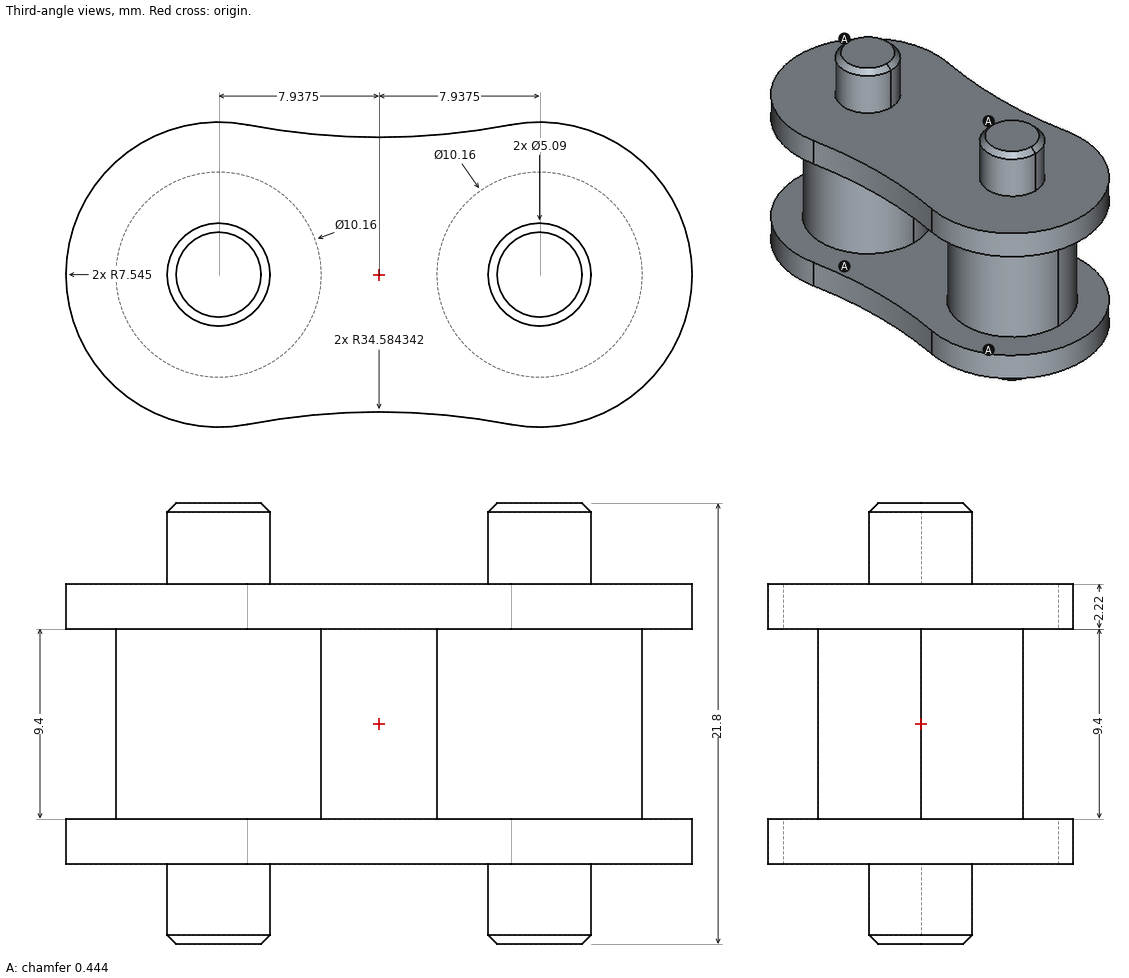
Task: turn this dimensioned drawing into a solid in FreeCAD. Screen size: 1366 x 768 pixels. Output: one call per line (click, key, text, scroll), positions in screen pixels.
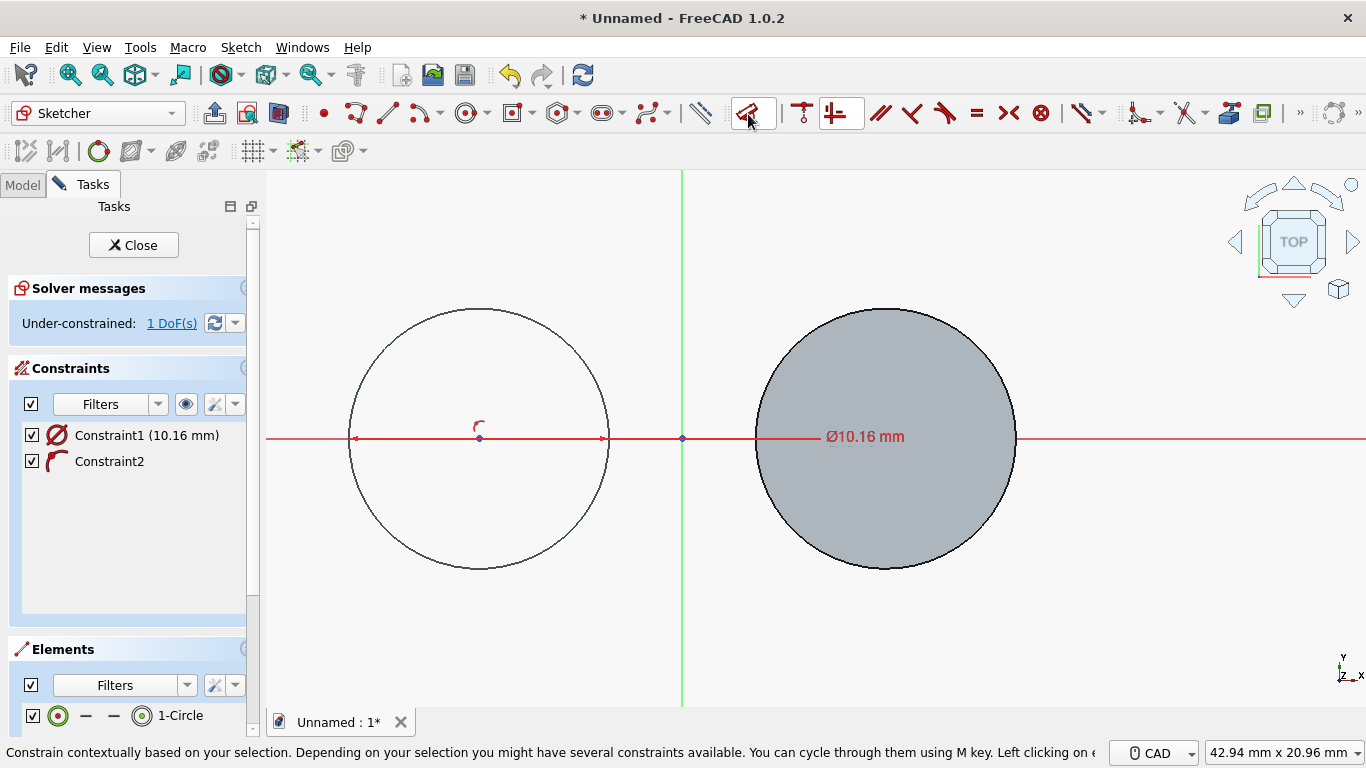
click(479, 439)
click(581, 473)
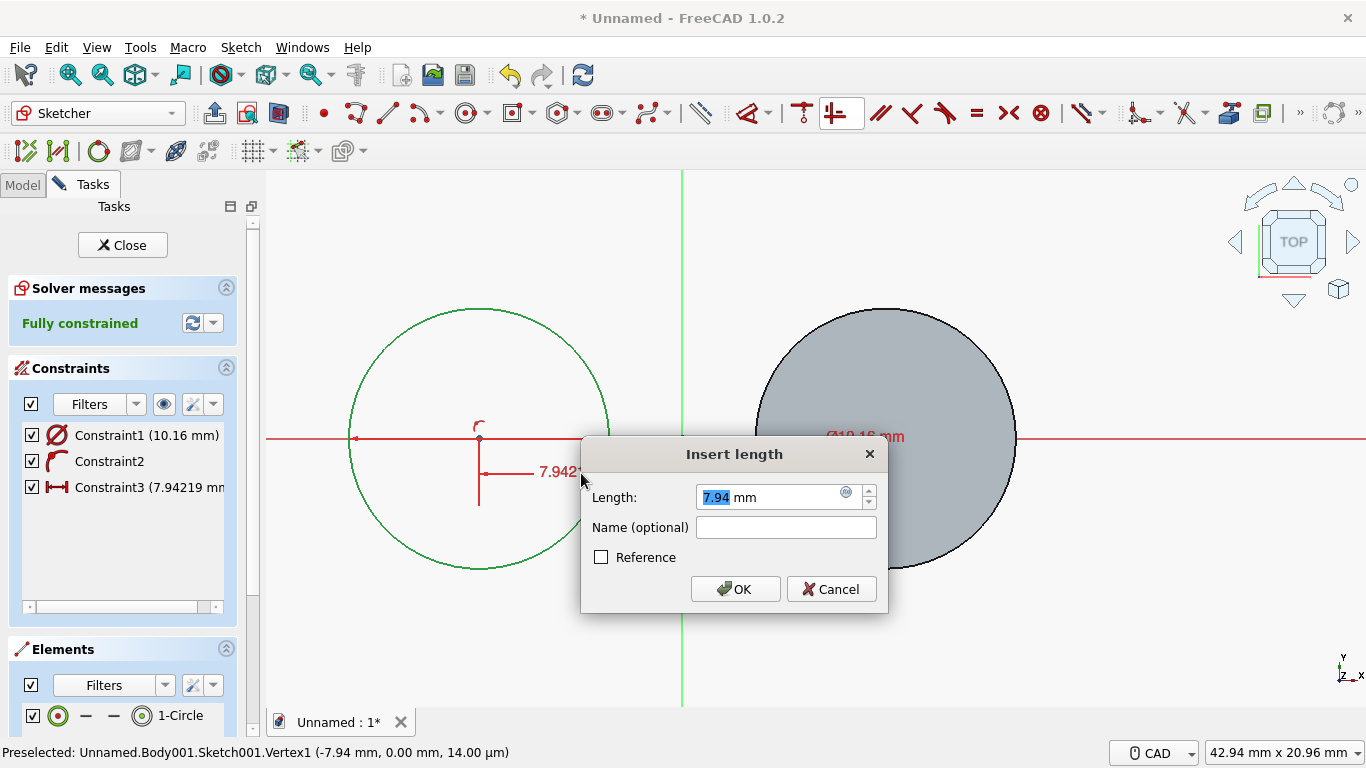
text(7.9375)
key(Return)
key(Escape)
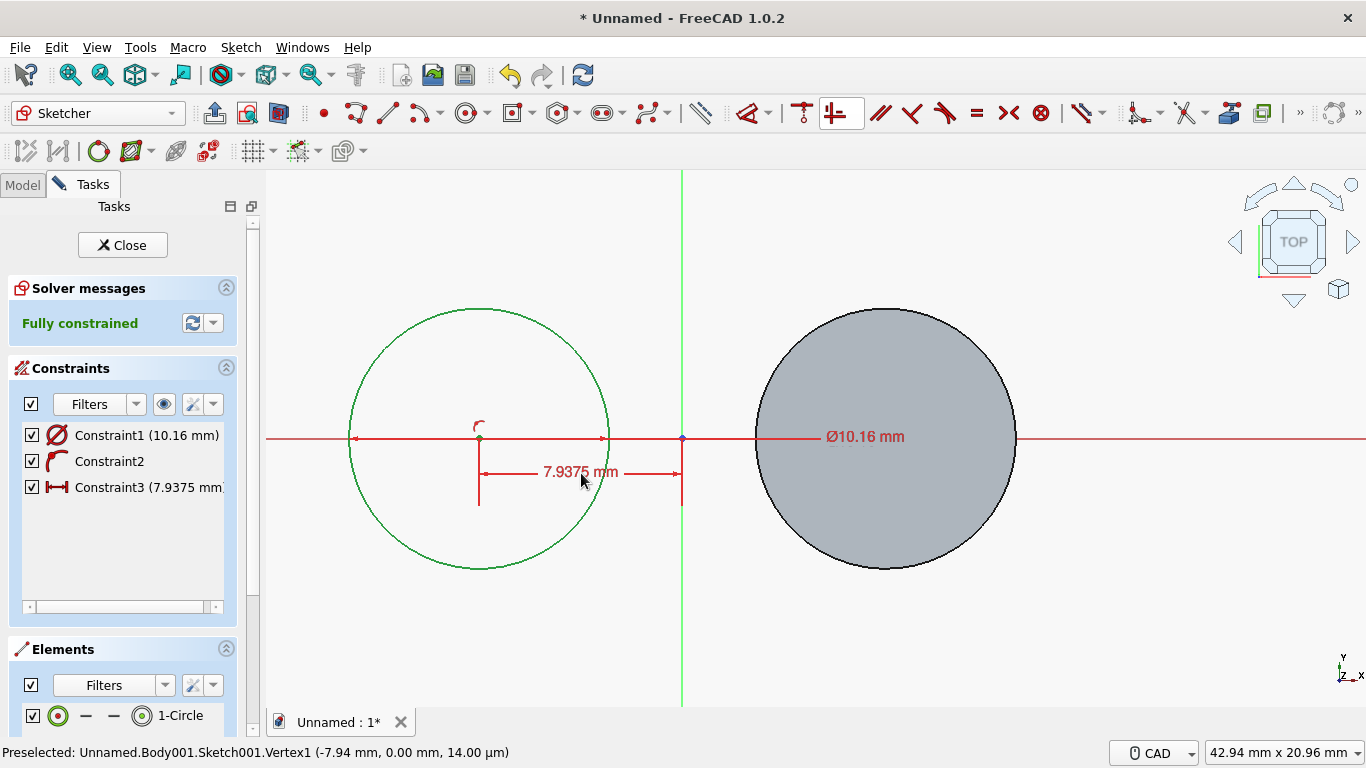
click(123, 245)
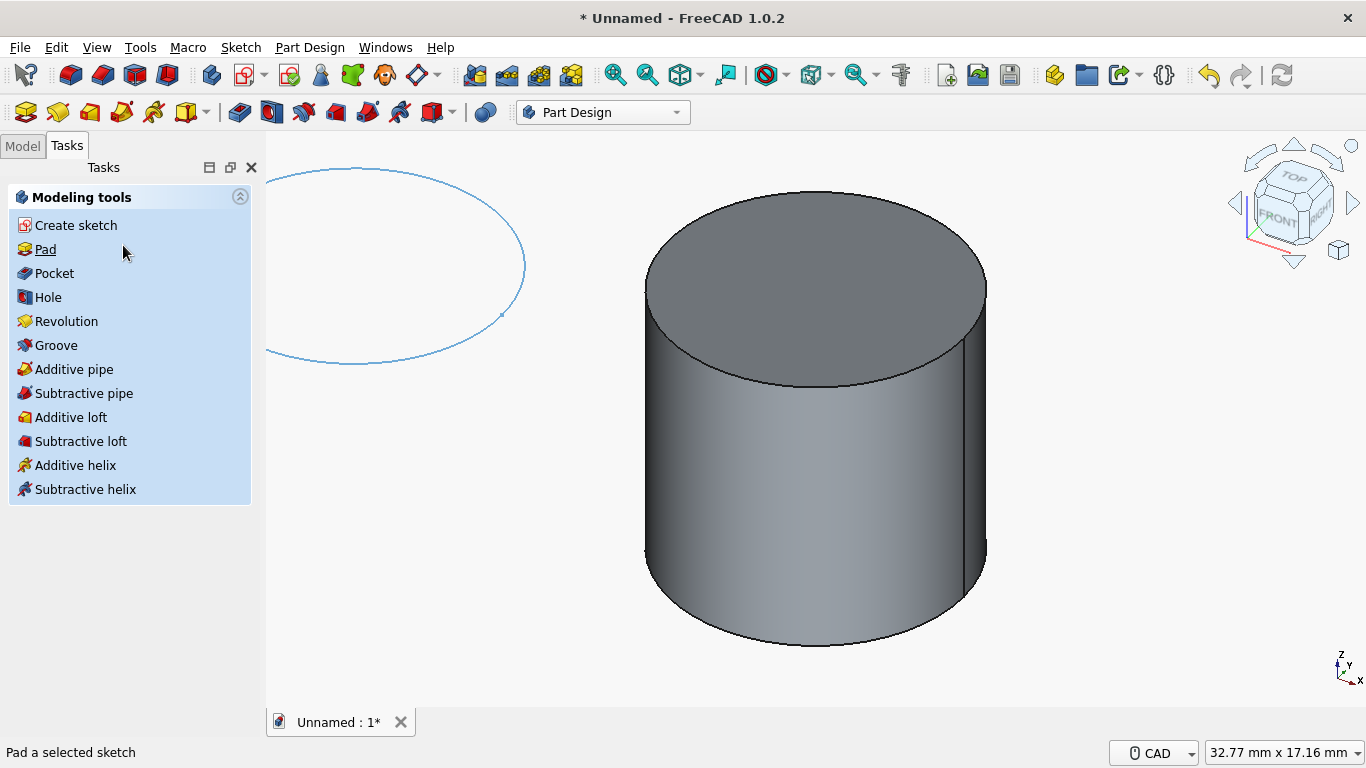
click(26, 112)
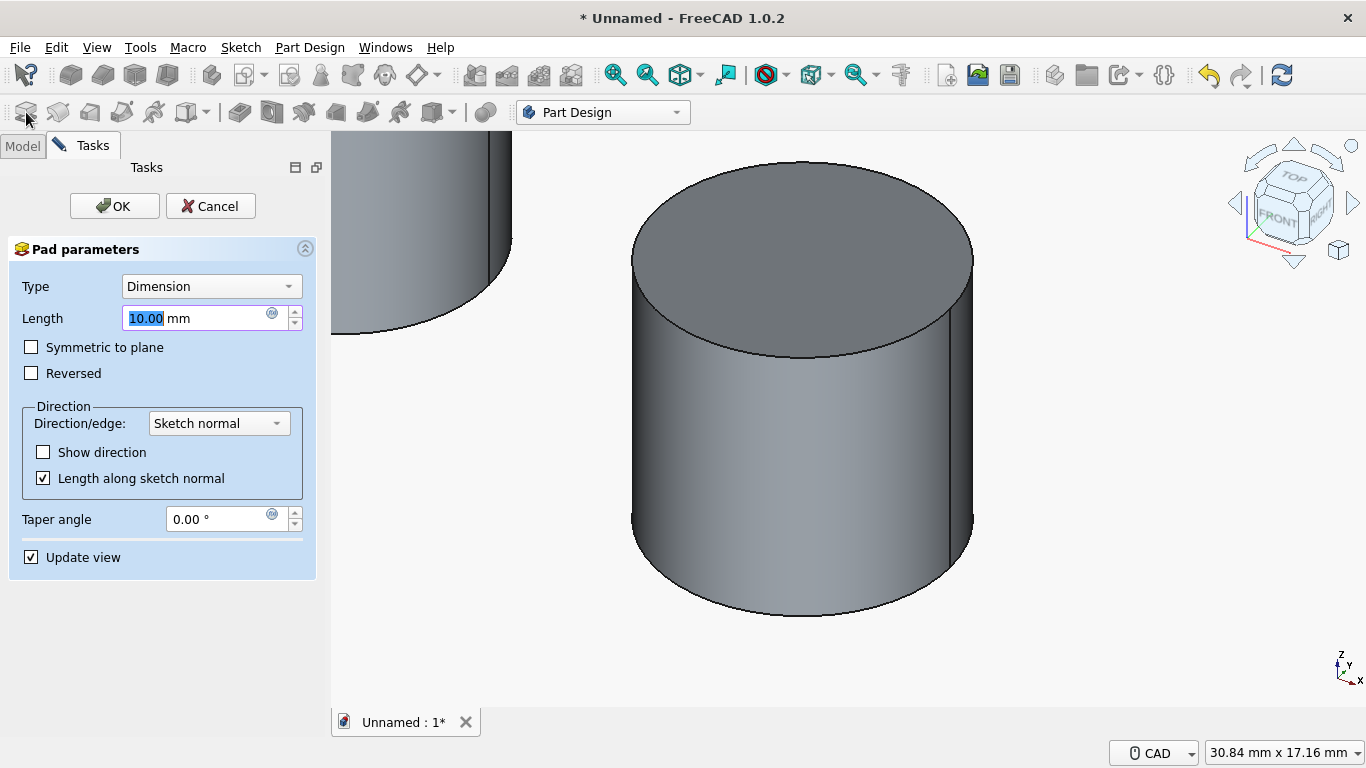
text(9.4)
key(Tab)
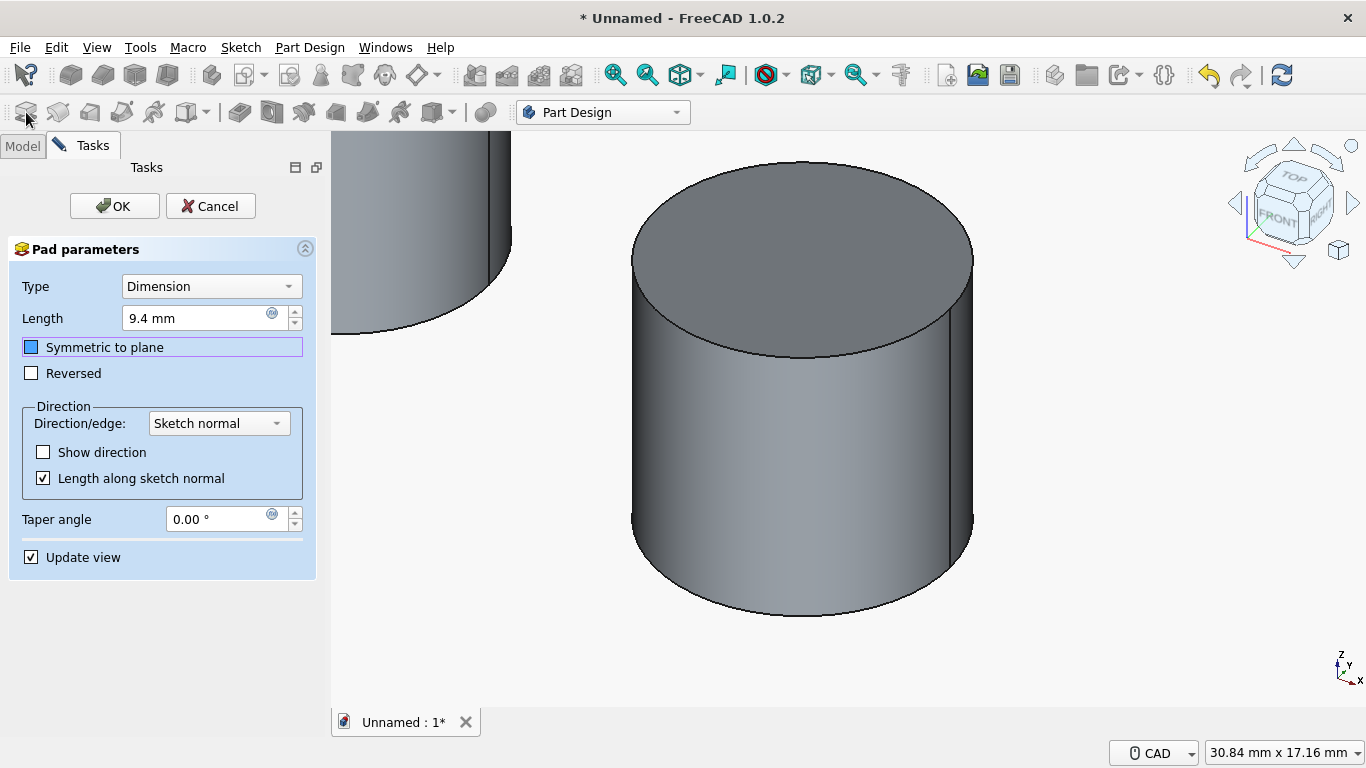
click(30, 347)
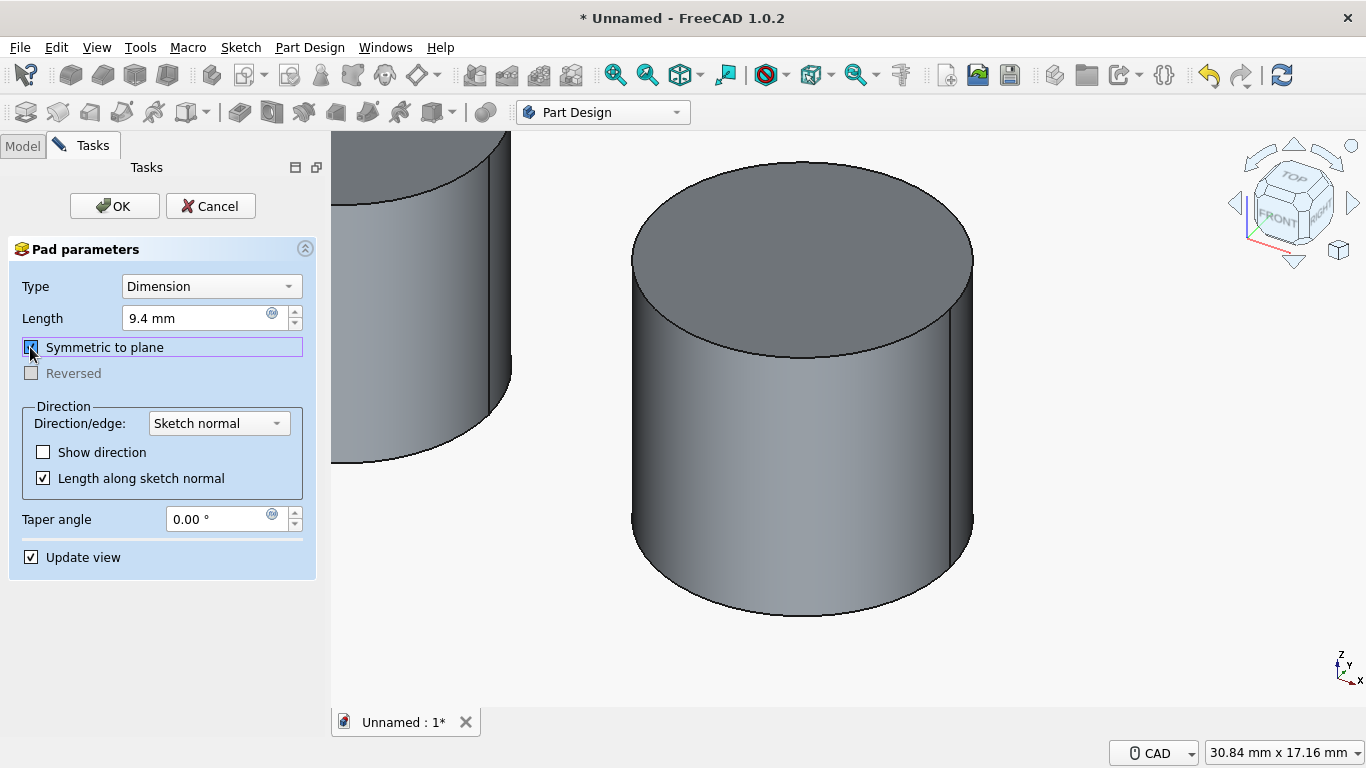
click(115, 206)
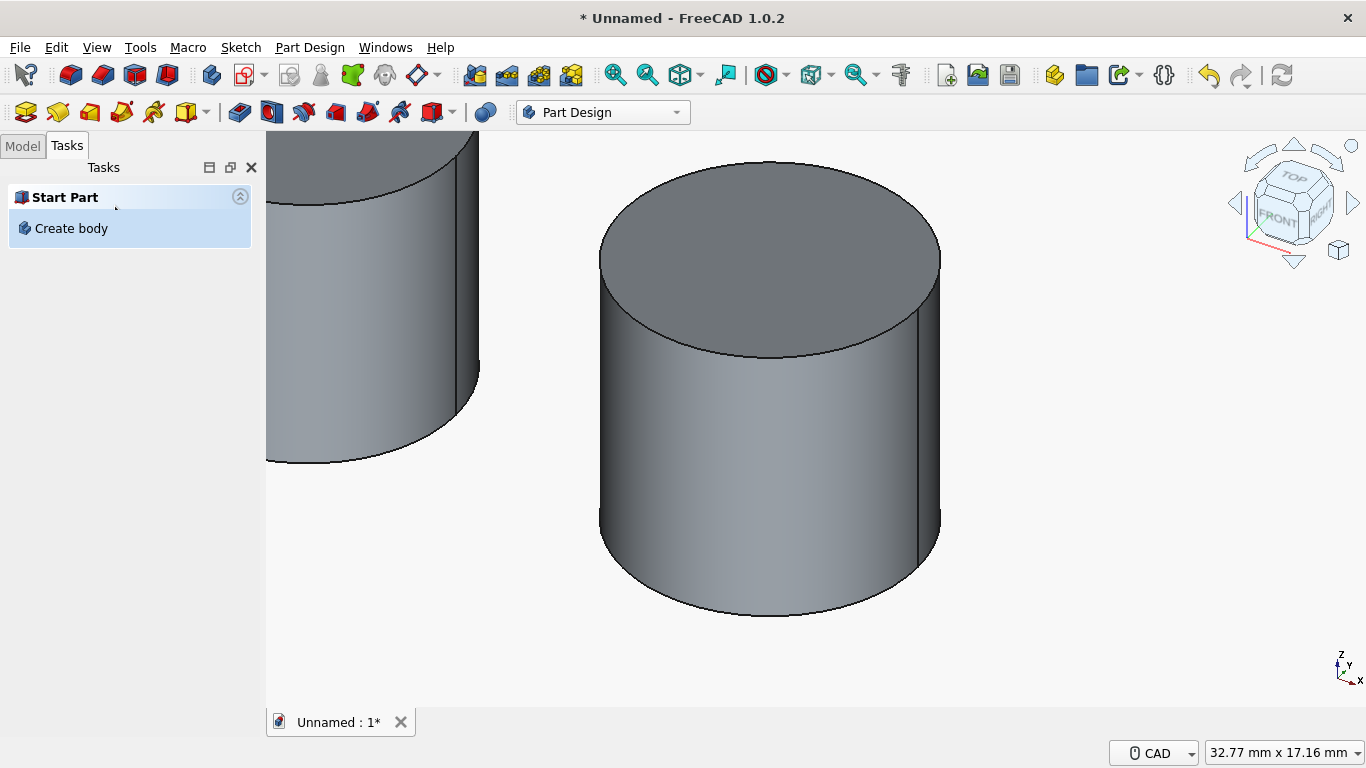
key(v)
key(f)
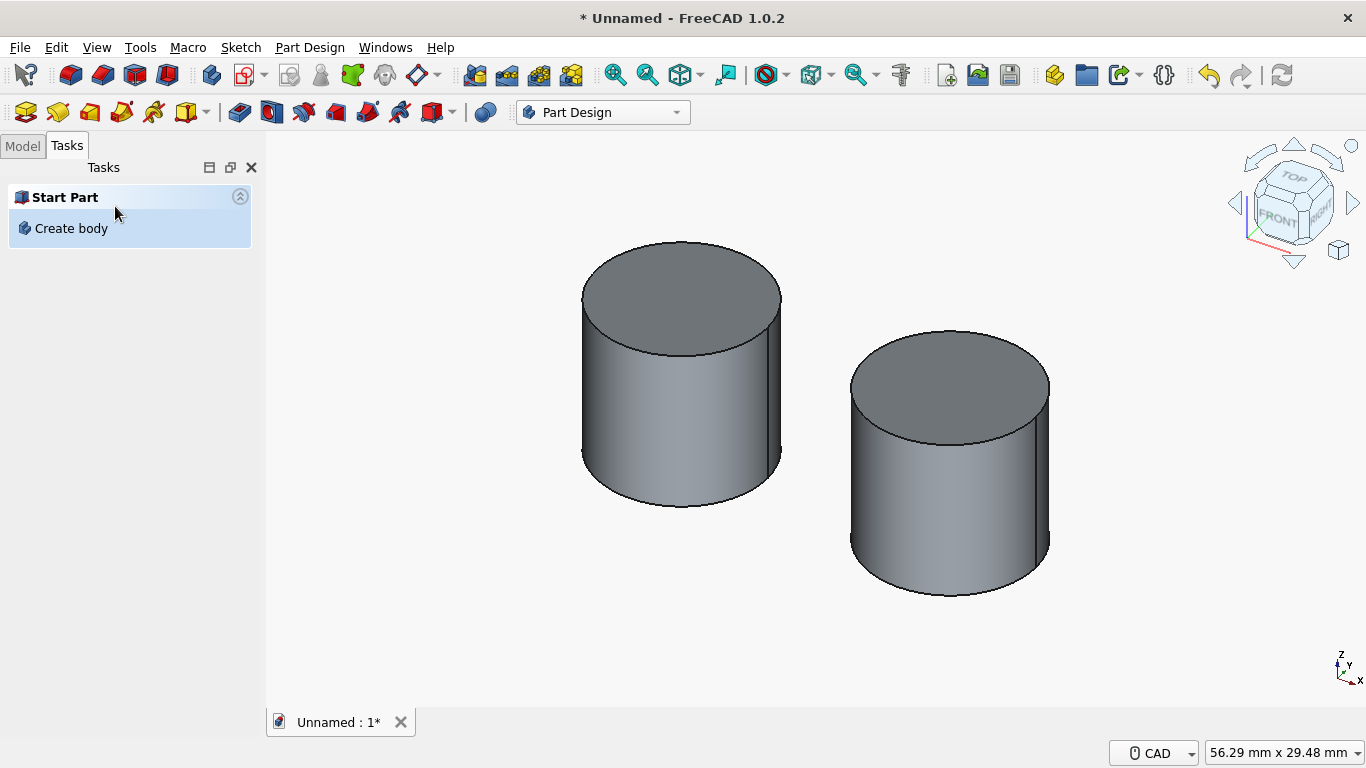
click(23, 145)